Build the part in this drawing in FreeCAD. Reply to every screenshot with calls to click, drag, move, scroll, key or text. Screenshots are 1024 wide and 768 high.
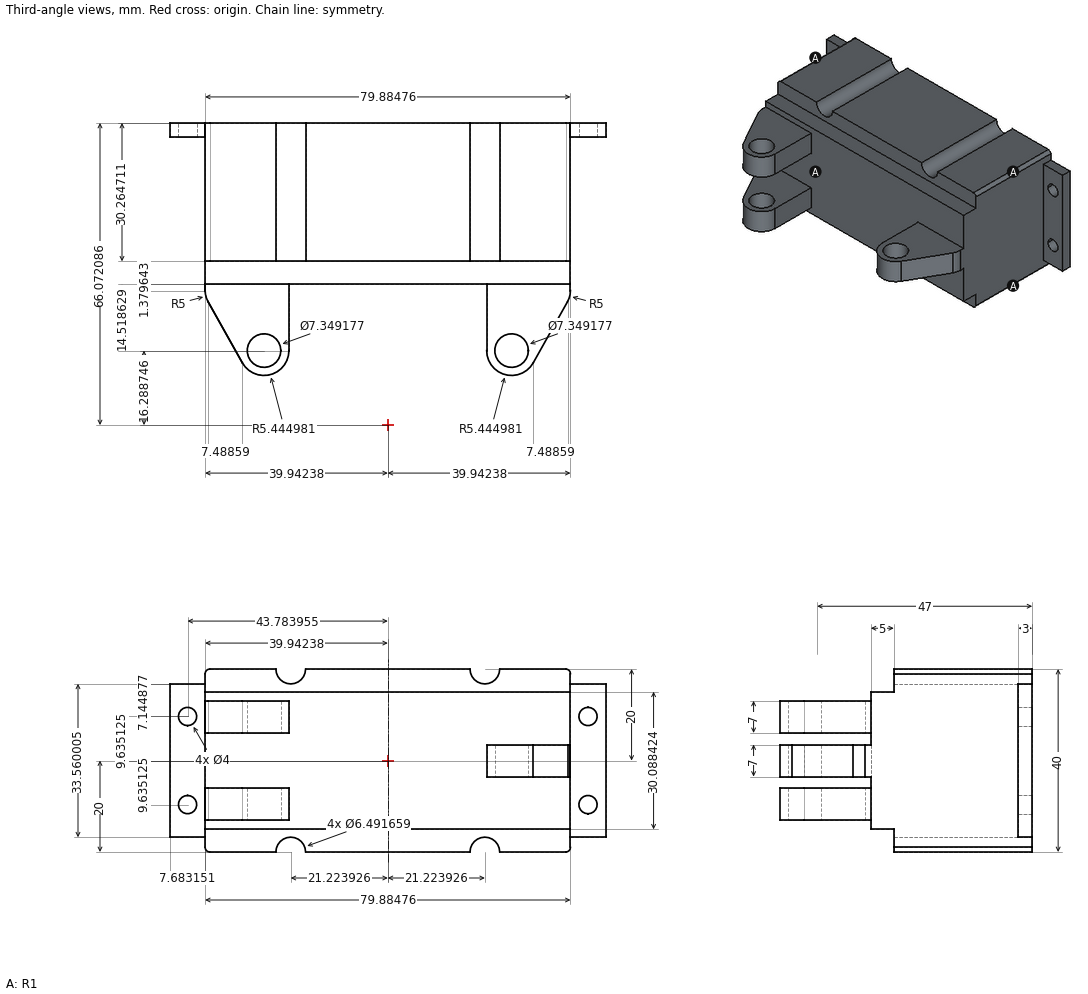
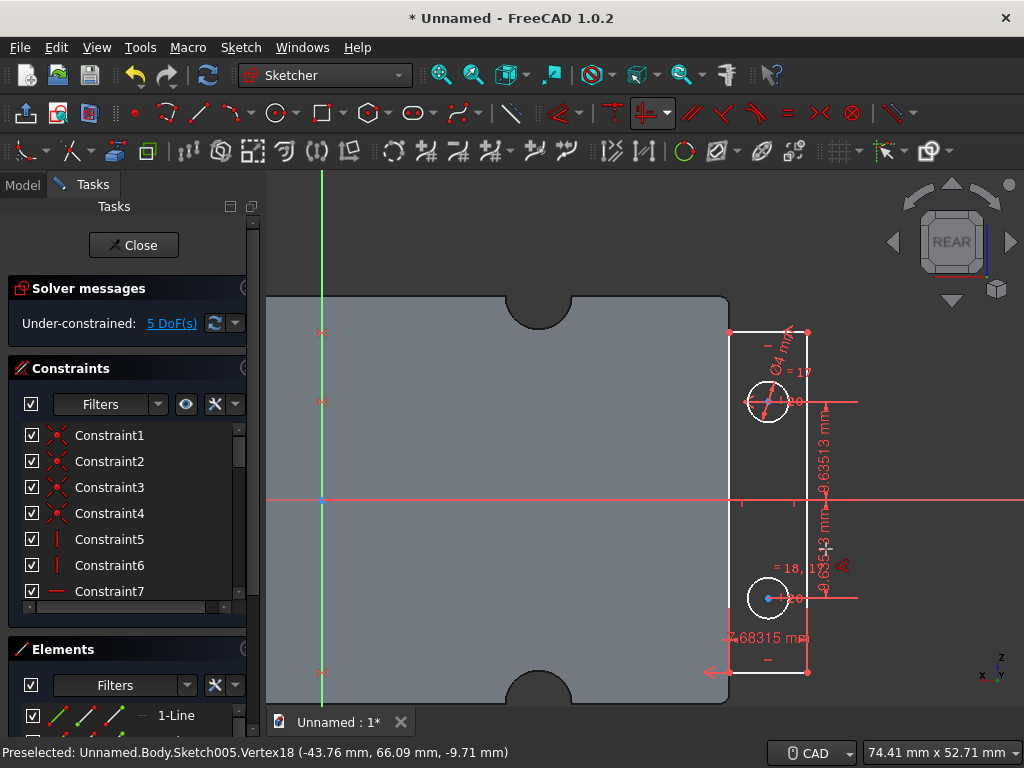
scroll(784, 388, down, 4)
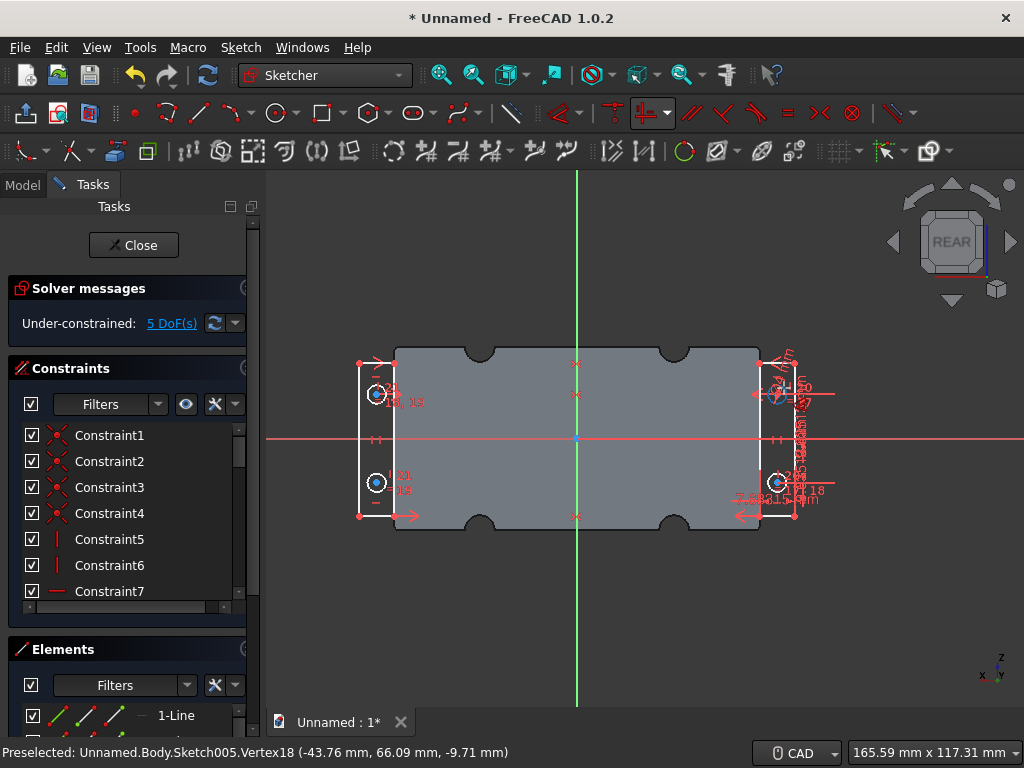
click(377, 483)
click(343, 461)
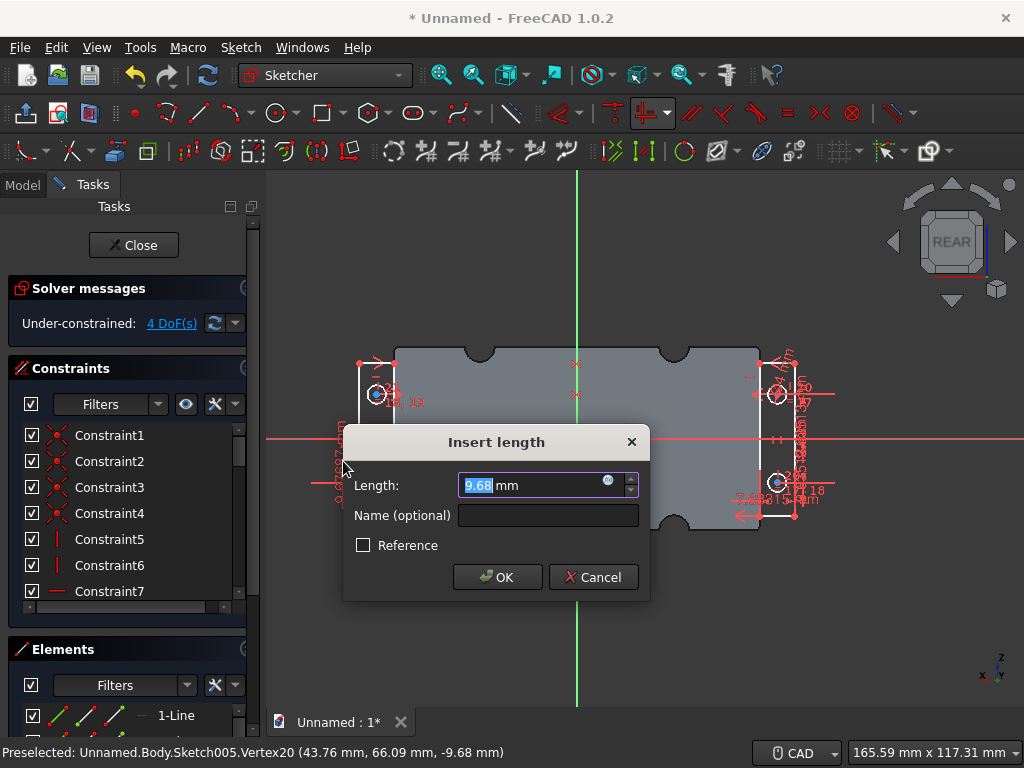
text(9.635125)
key(Return)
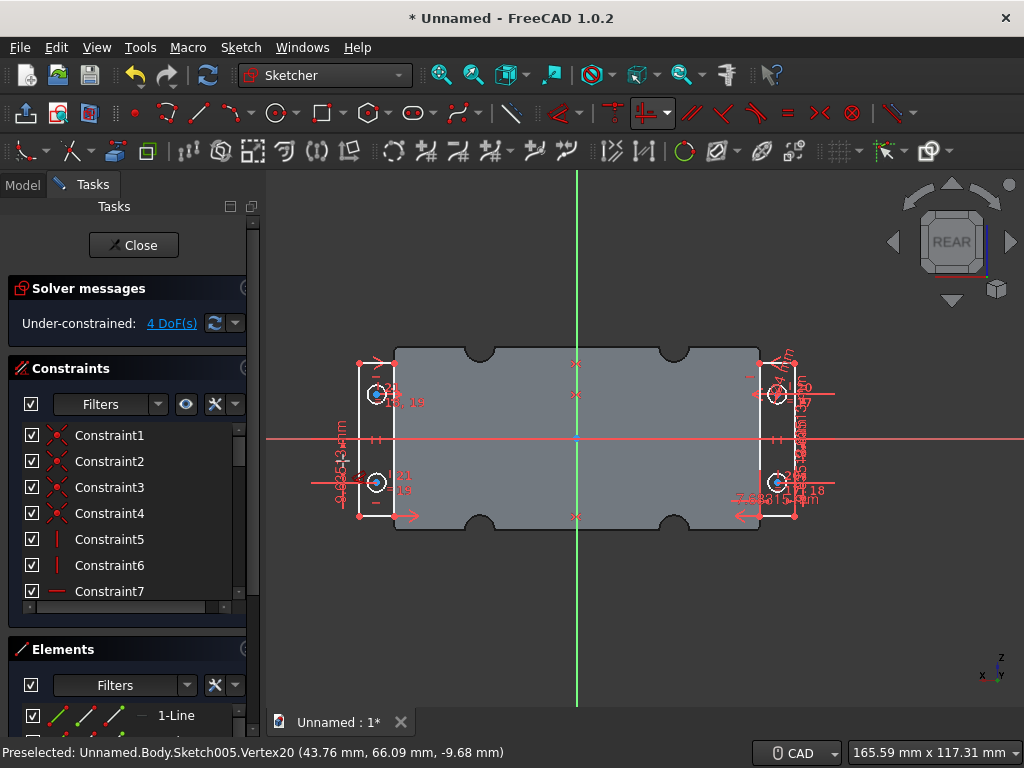
click(760, 409)
click(726, 404)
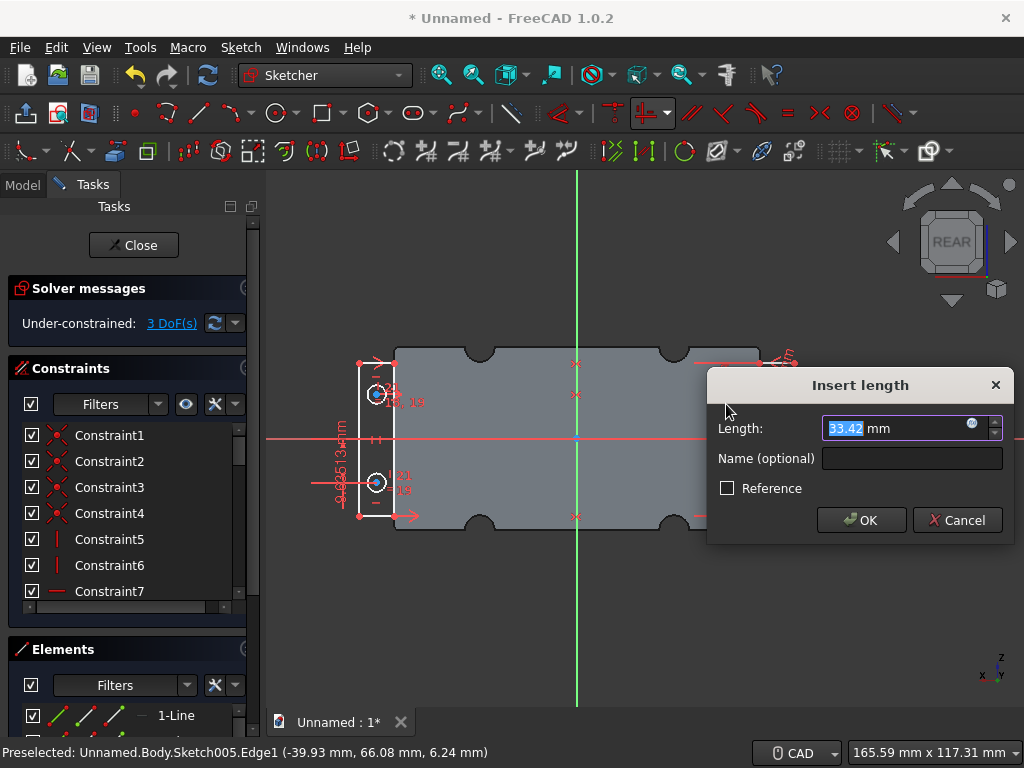
text(33.560005)
key(Return)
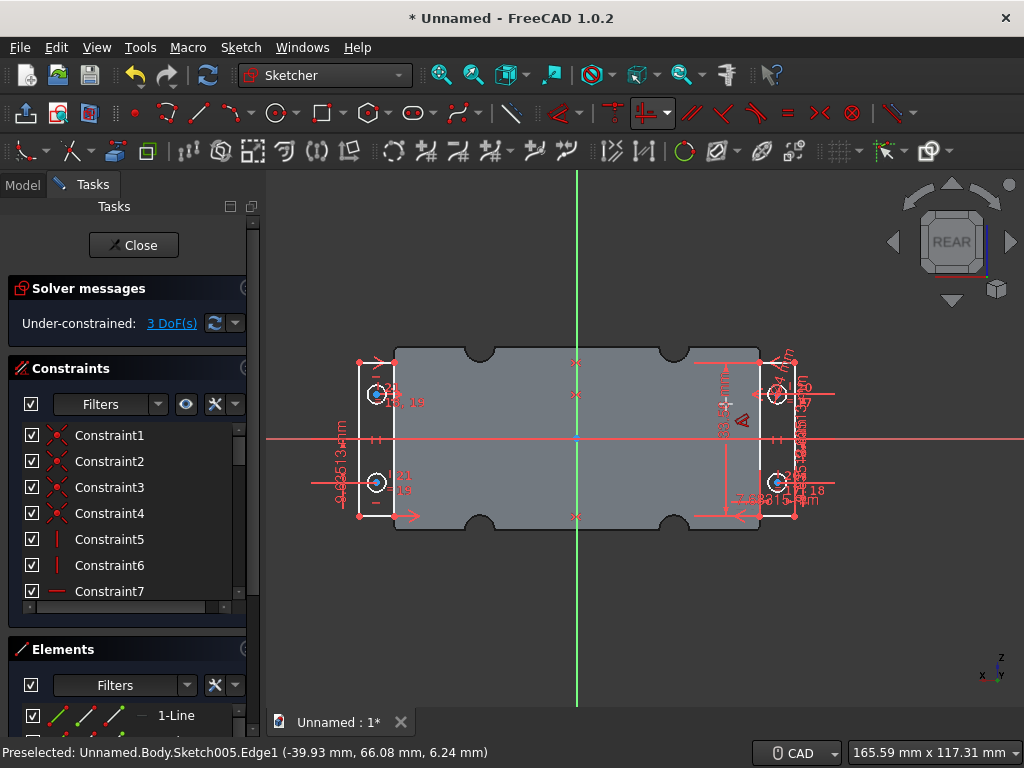
click(760, 363)
click(668, 329)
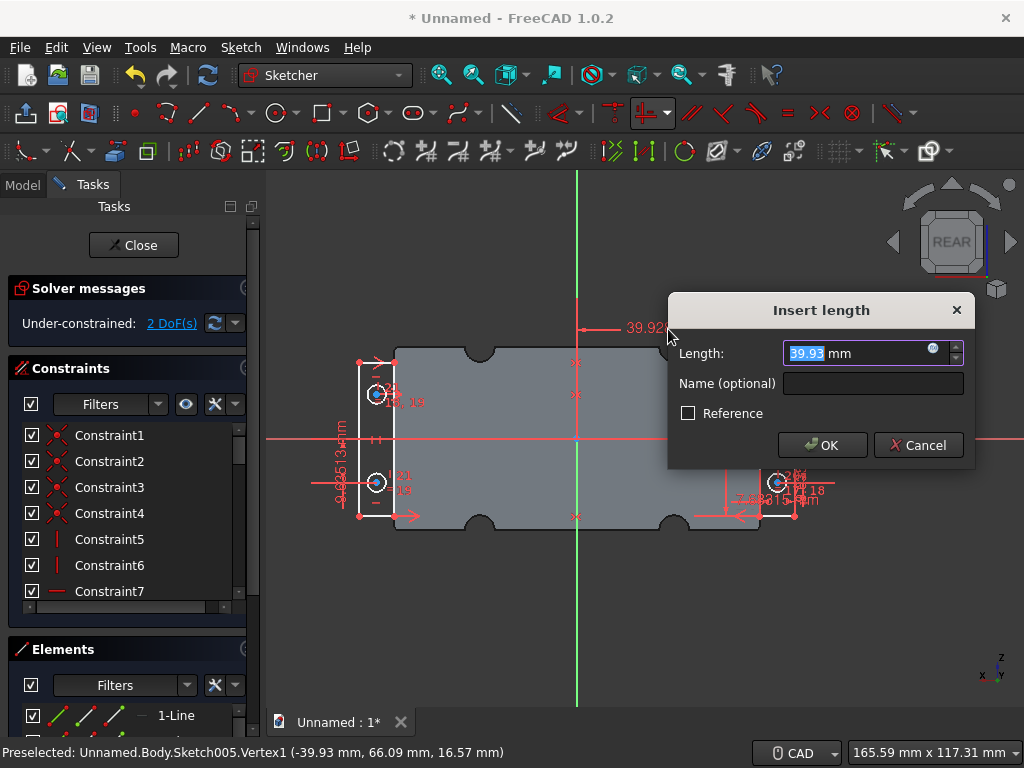
text(39.94238)
key(Return)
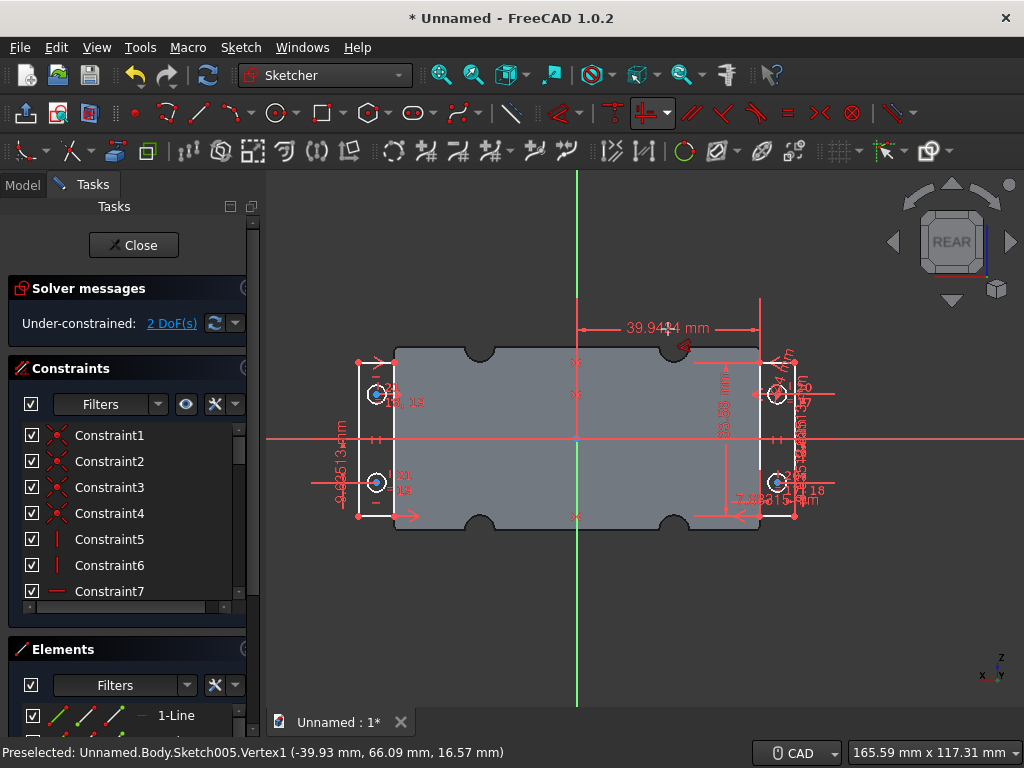
click(777, 394)
click(677, 360)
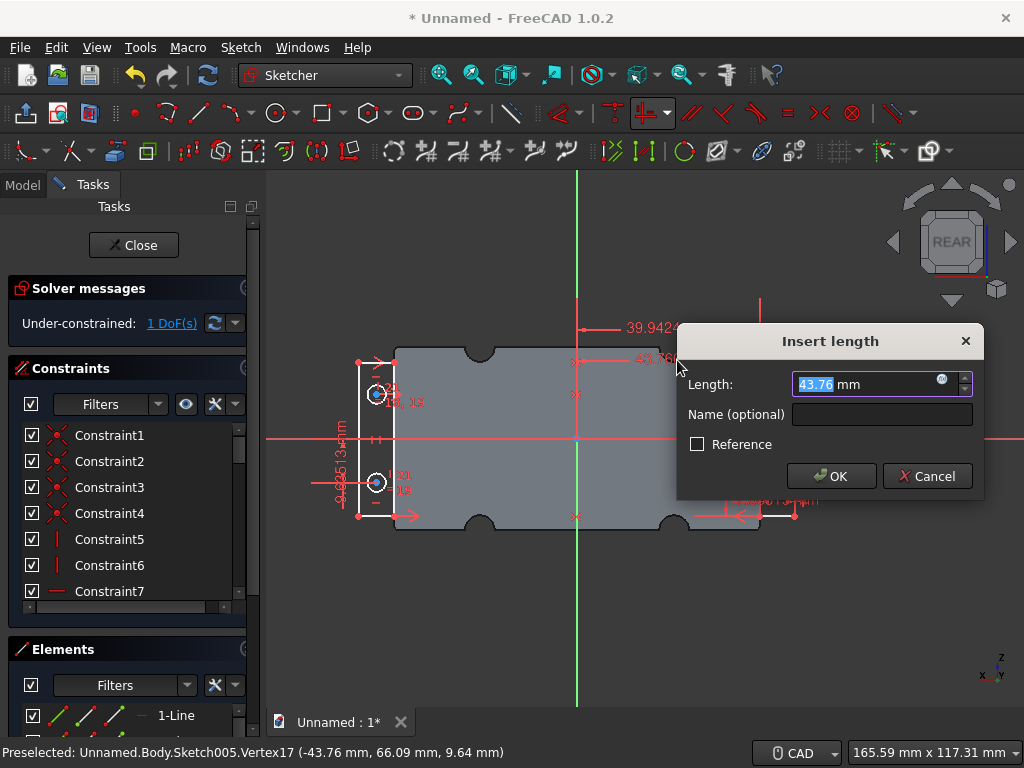
text(43.783955)
key(Return)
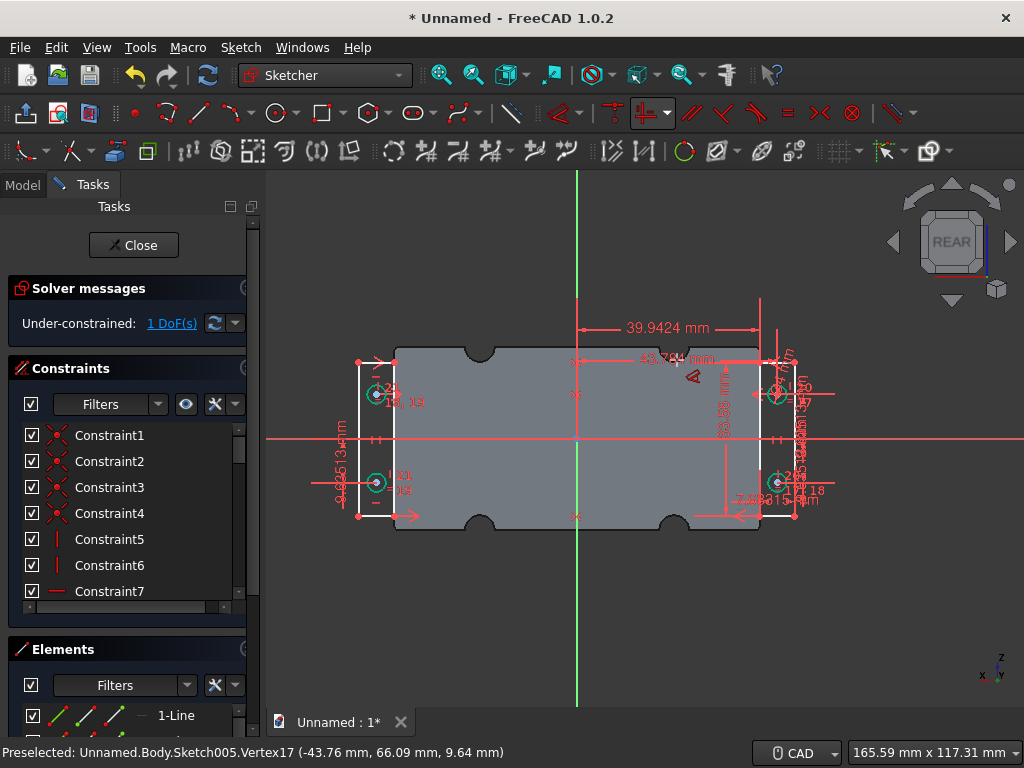
click(795, 363)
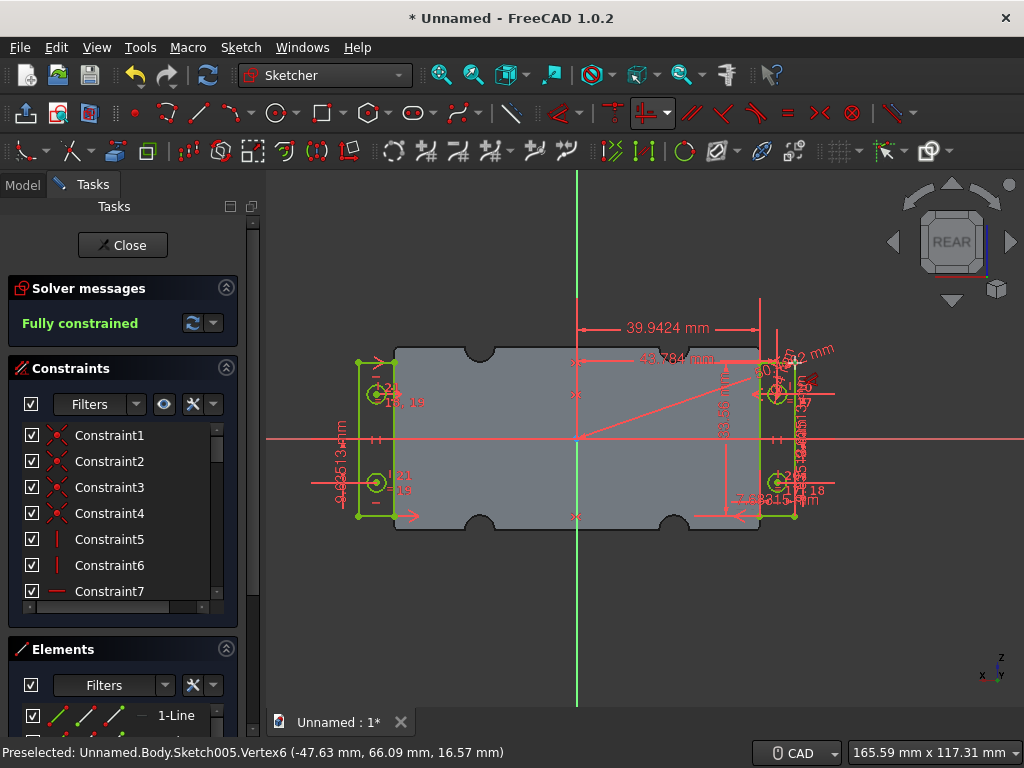
click(777, 394)
click(647, 386)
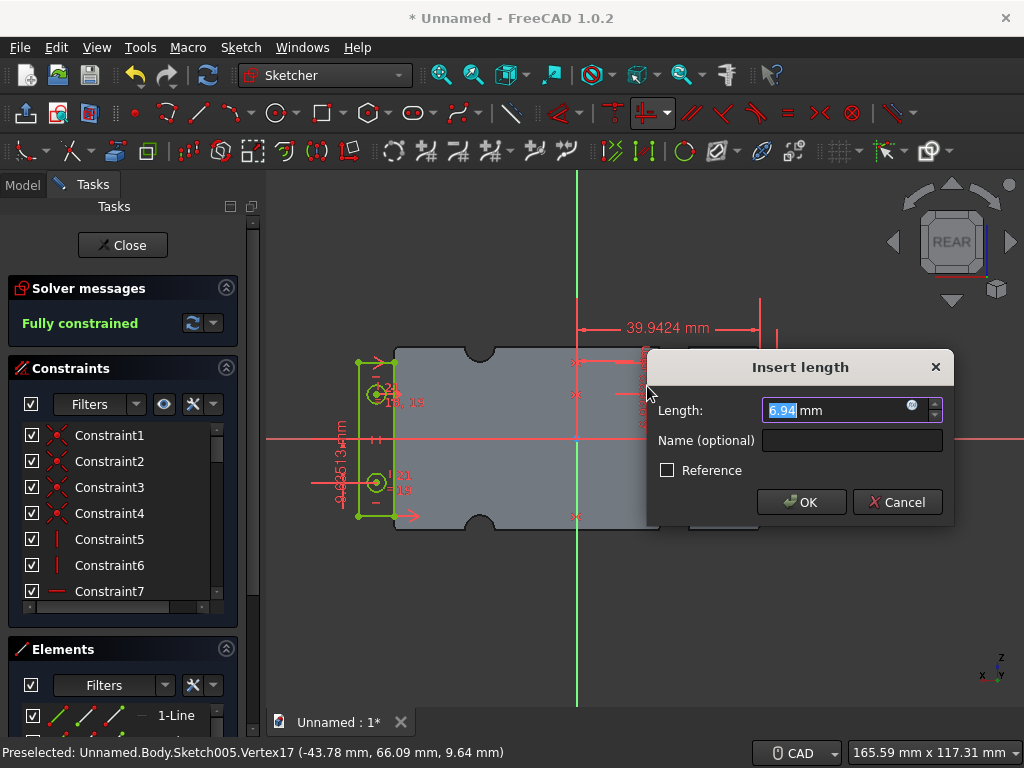
text(7.144877)
key(Return)
key(Escape)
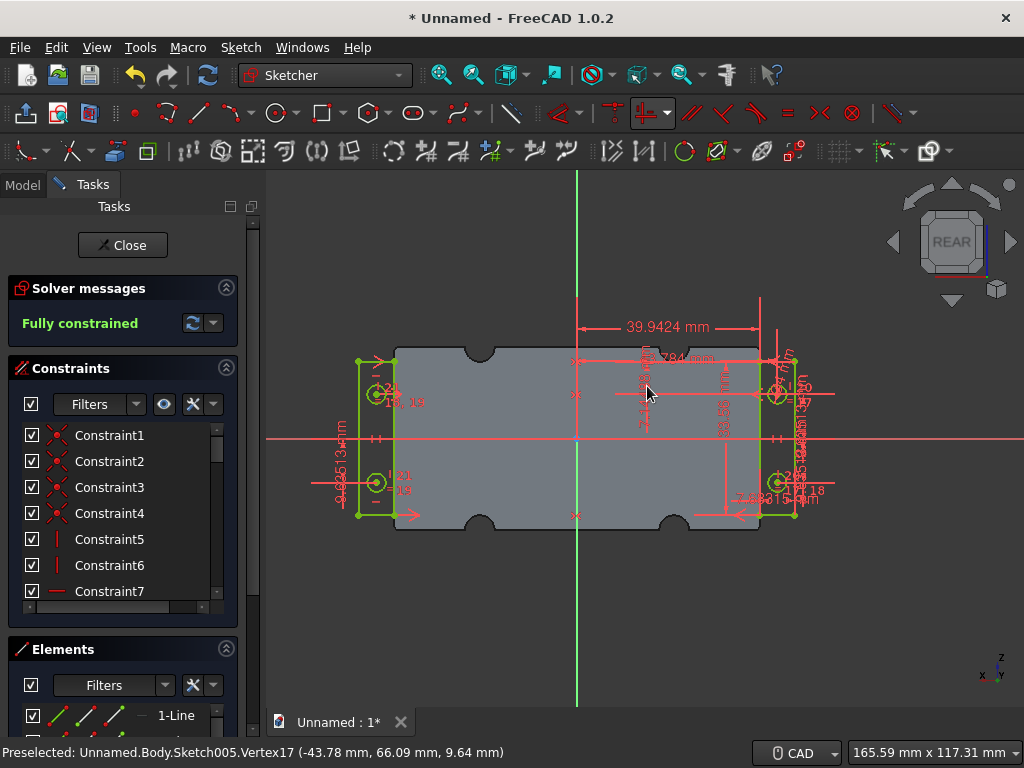
click(123, 245)